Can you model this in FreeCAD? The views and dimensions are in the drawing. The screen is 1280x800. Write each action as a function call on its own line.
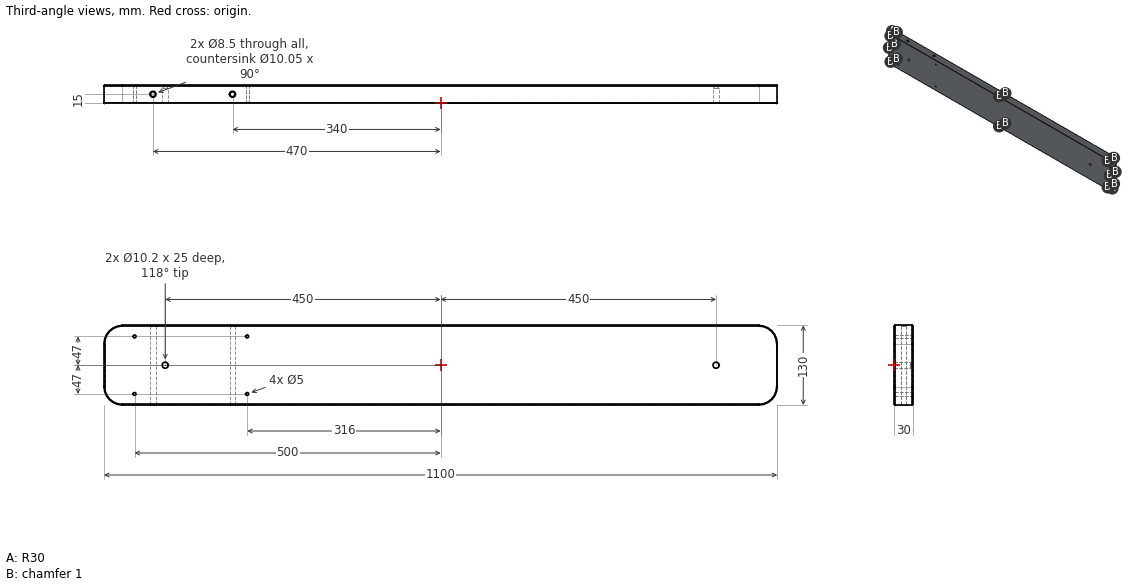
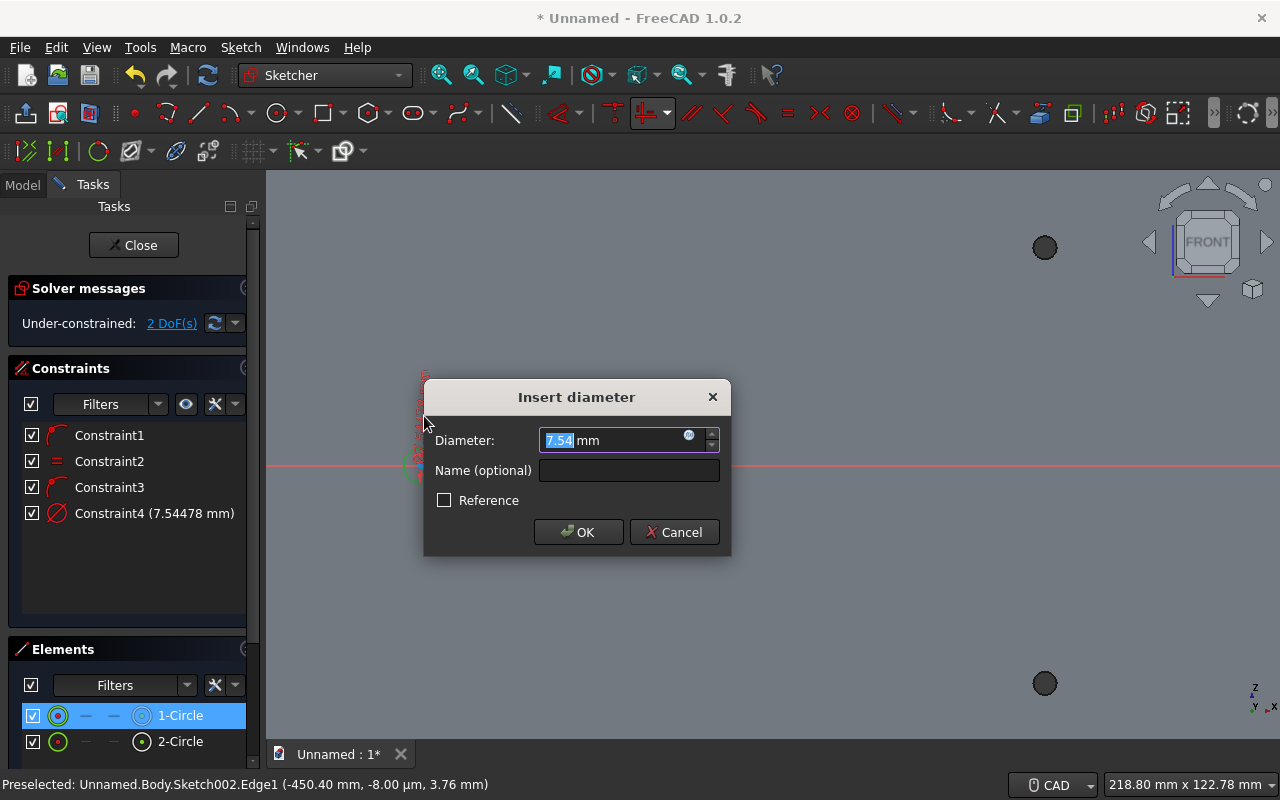
text(10.2)
key(Return)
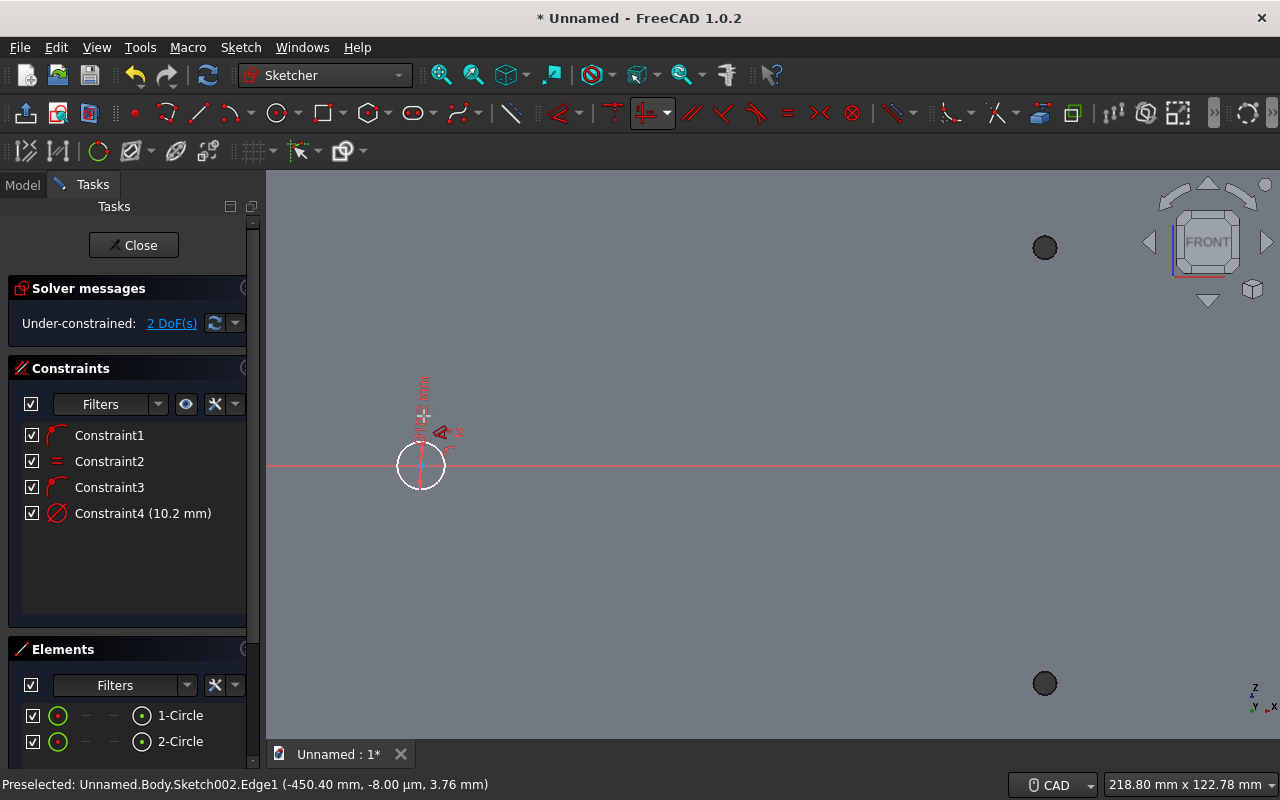
scroll(422, 453, down, 10)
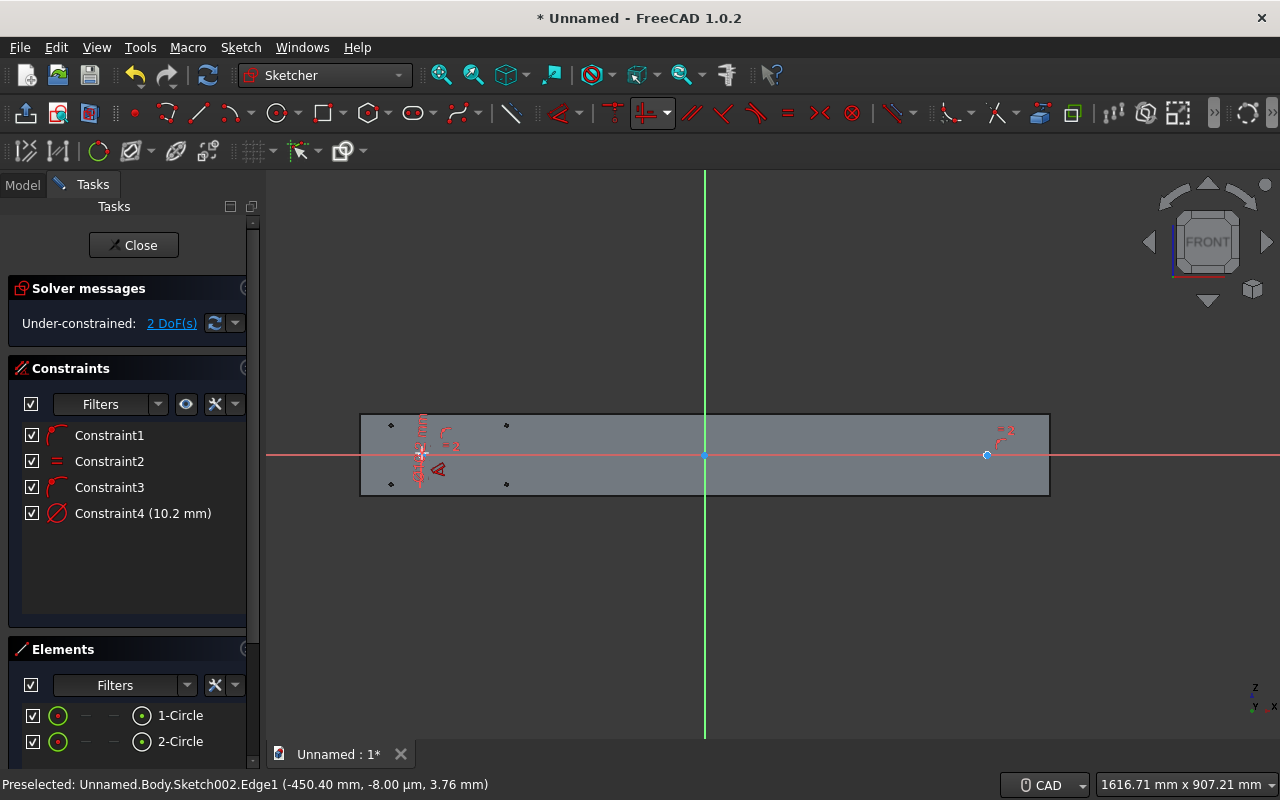
click(422, 455)
click(563, 489)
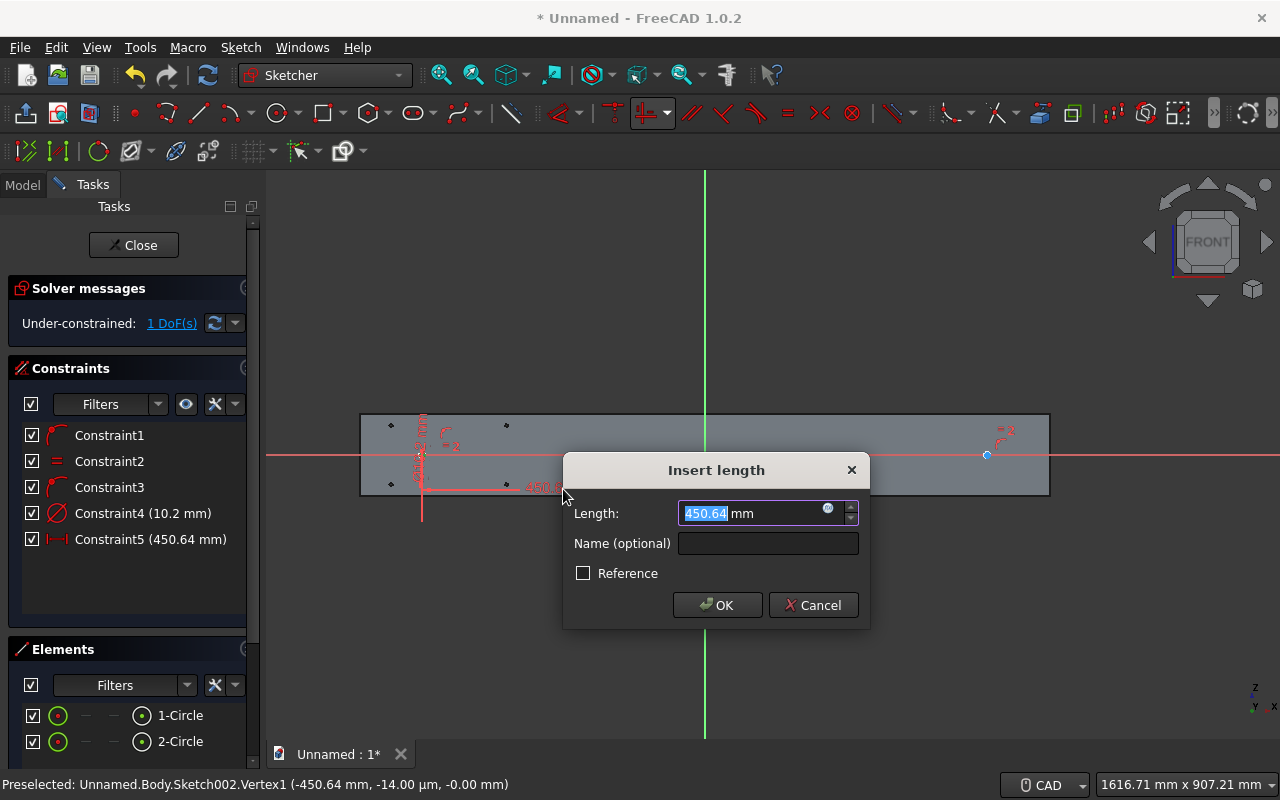
text(450)
key(Return)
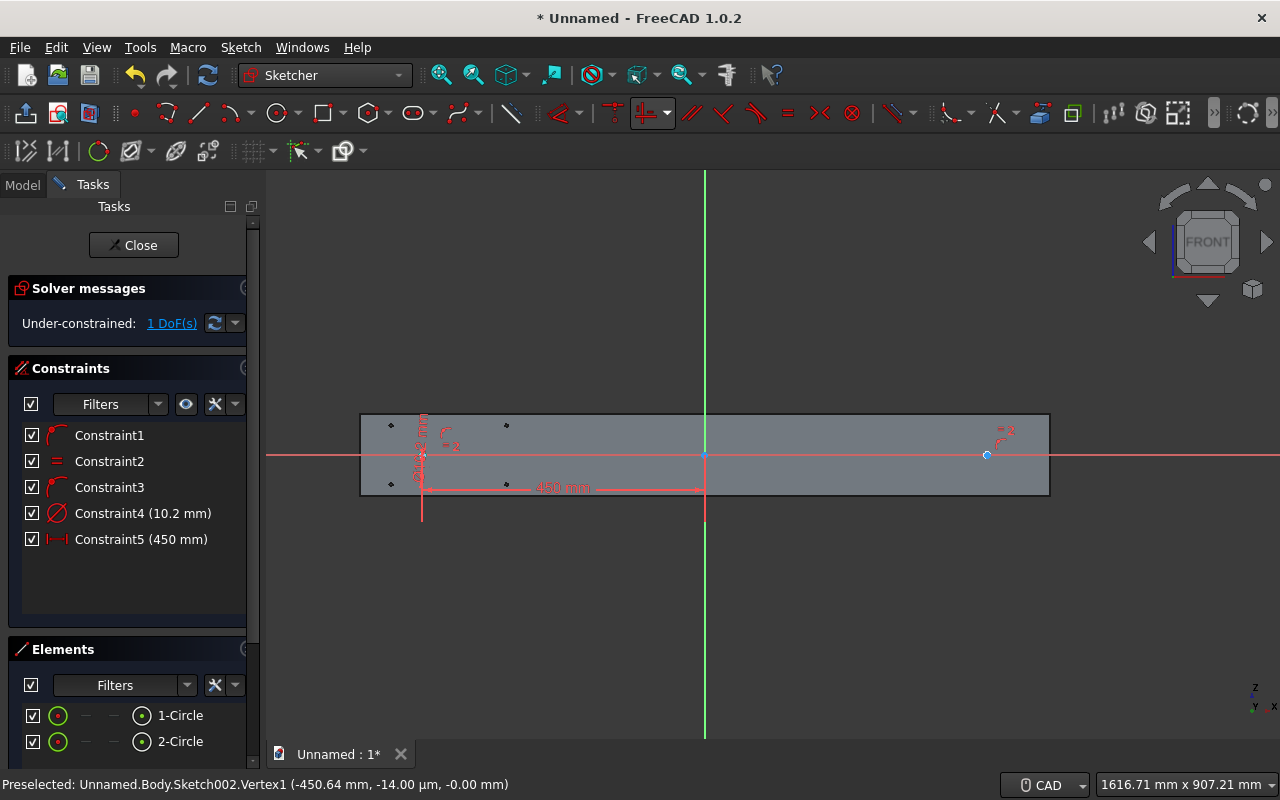
click(987, 455)
click(846, 489)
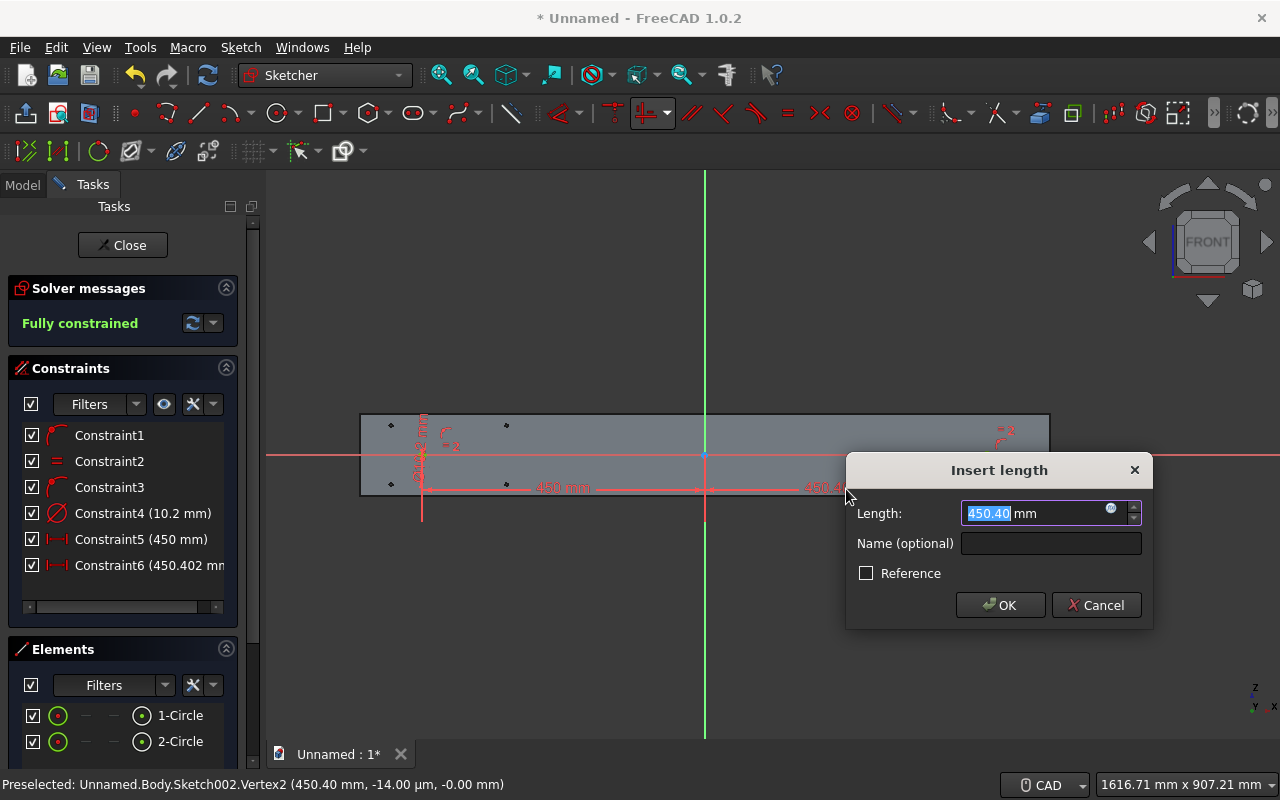
text(450)
key(Return)
key(Escape)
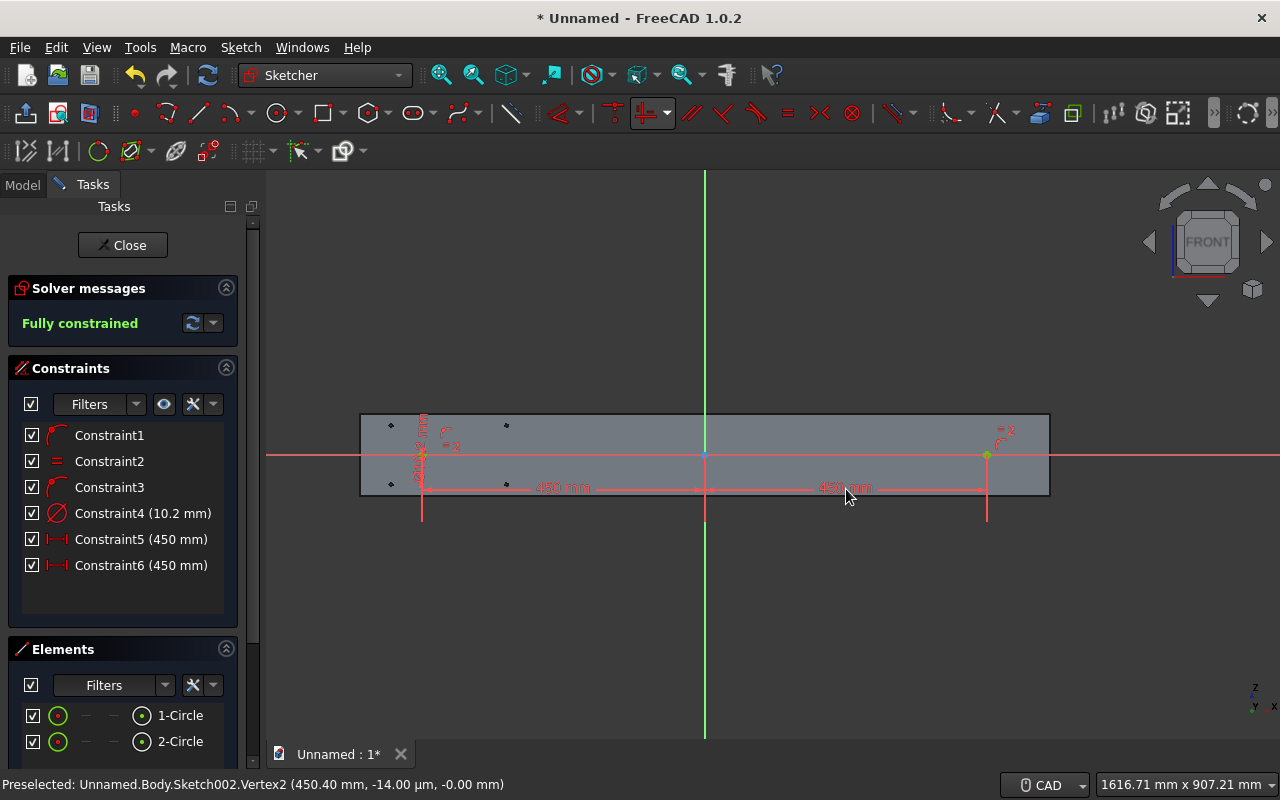
click(123, 245)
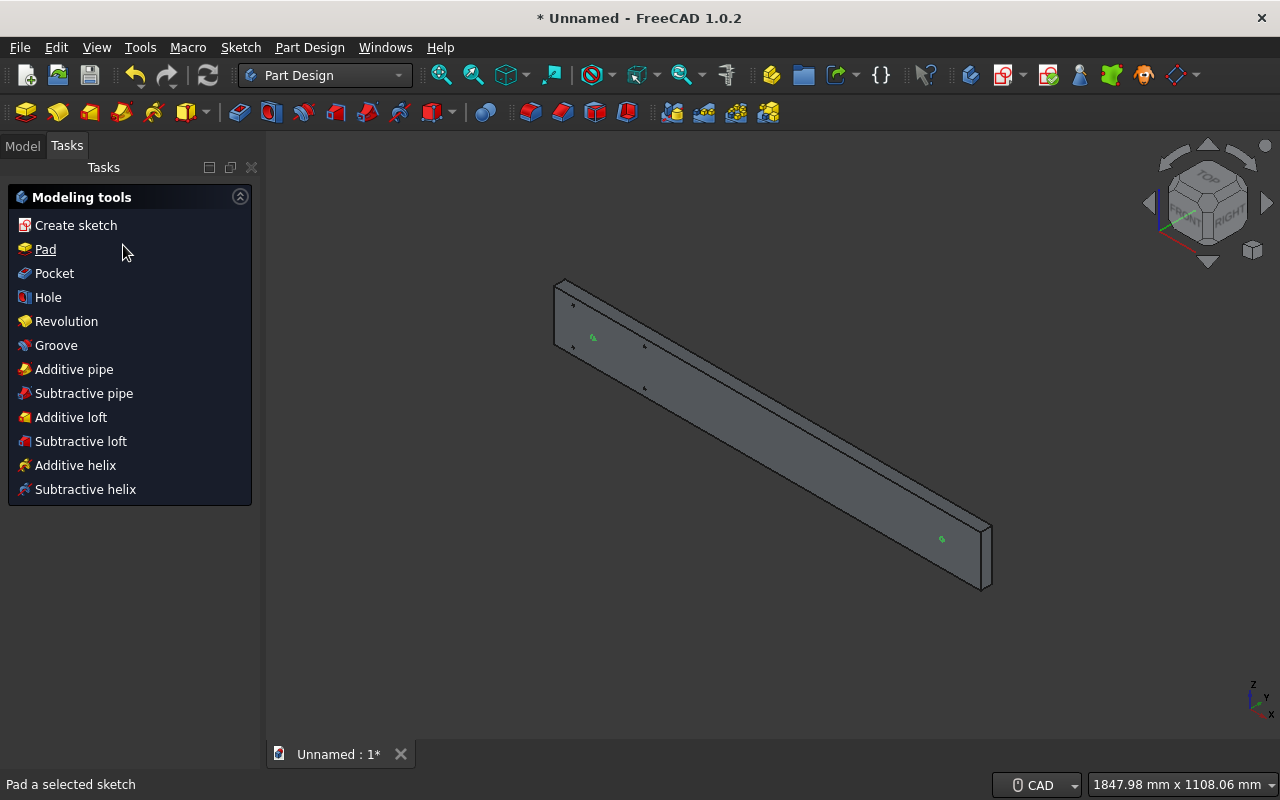
click(272, 112)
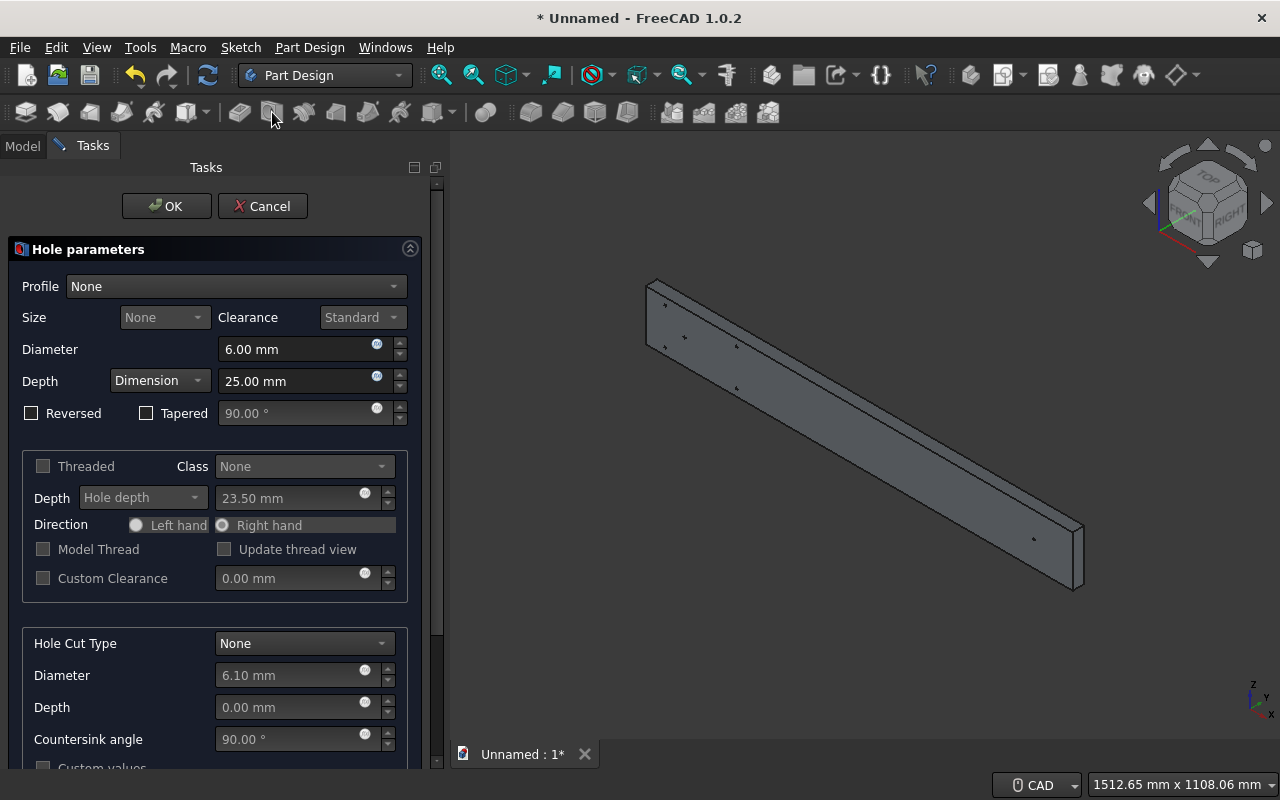
triple_click(305, 349)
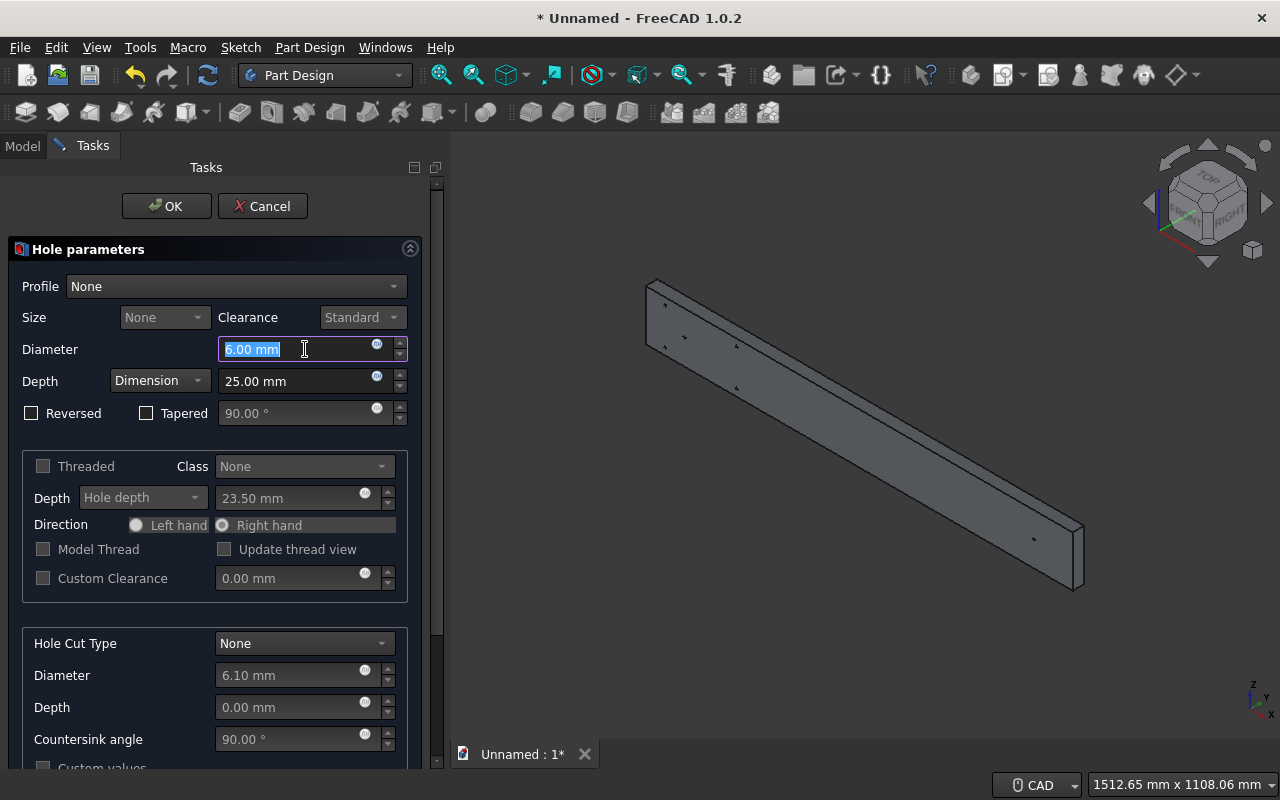
text(10.2)
key(Tab)